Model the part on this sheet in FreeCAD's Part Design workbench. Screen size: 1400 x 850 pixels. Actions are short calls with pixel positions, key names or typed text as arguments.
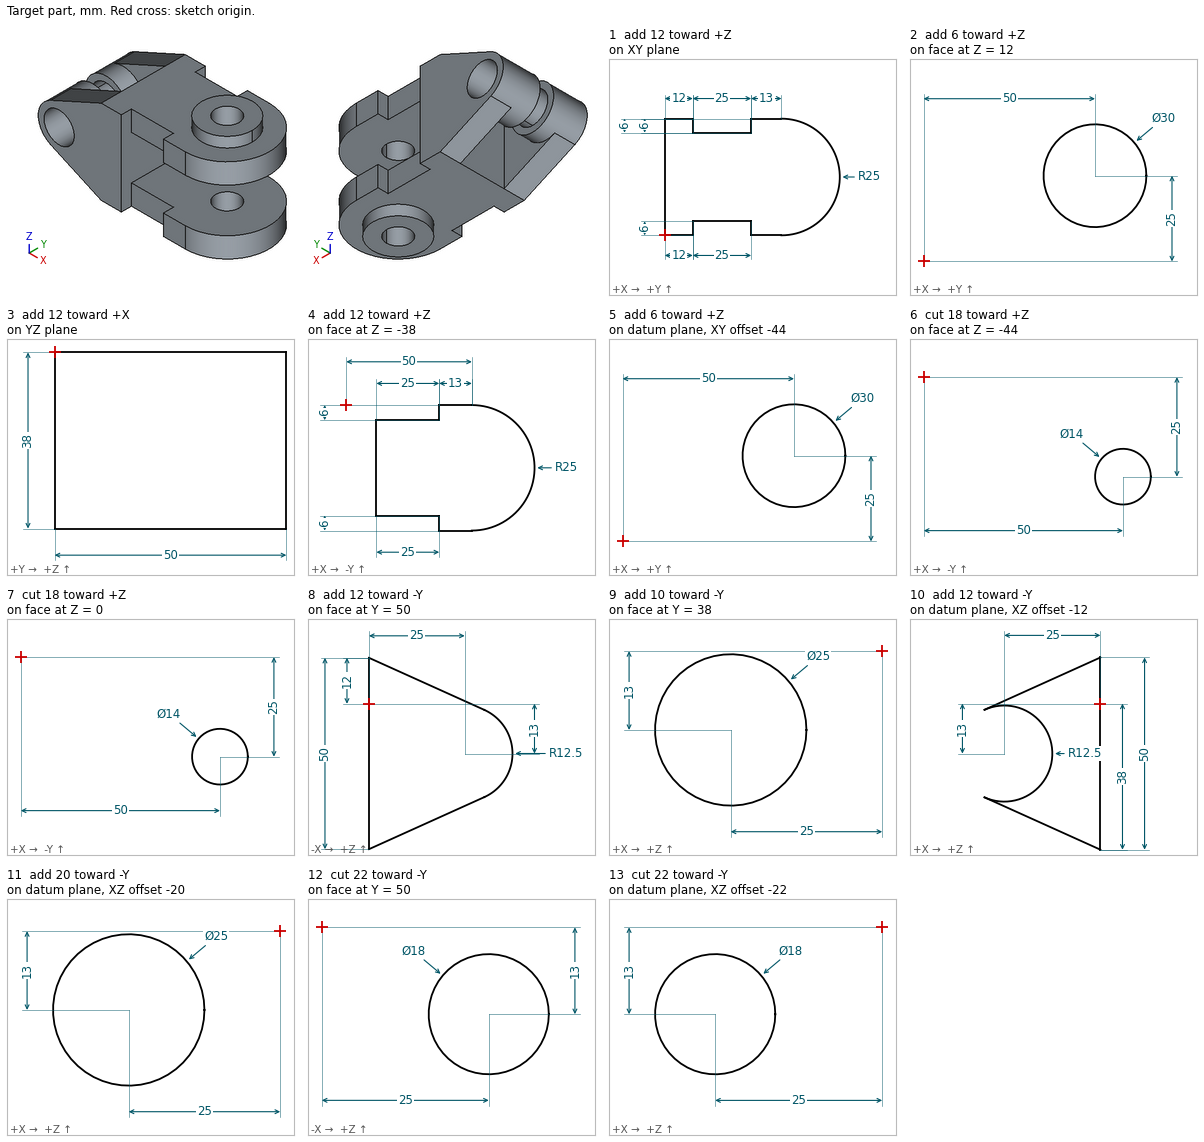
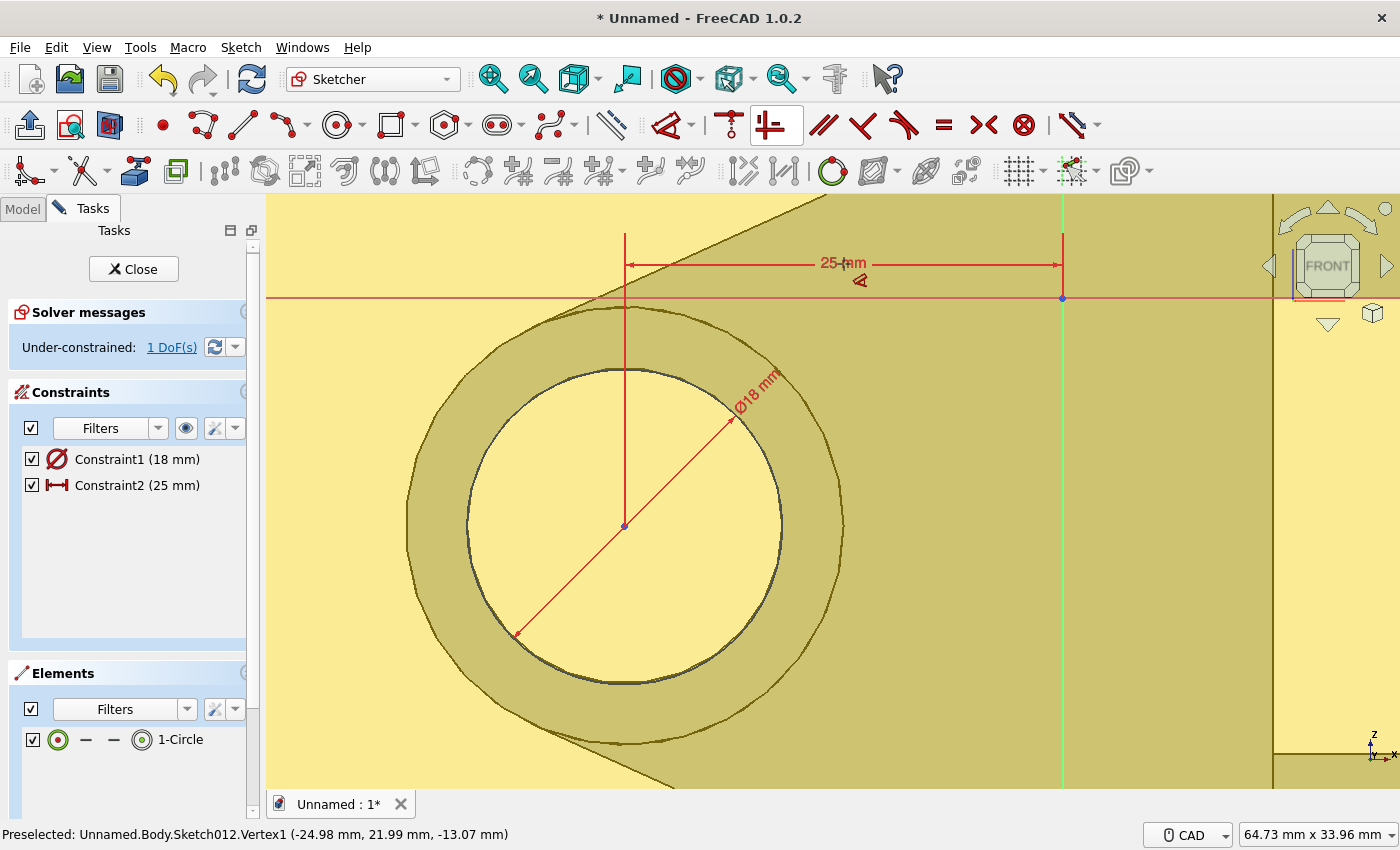
click(625, 527)
click(1097, 413)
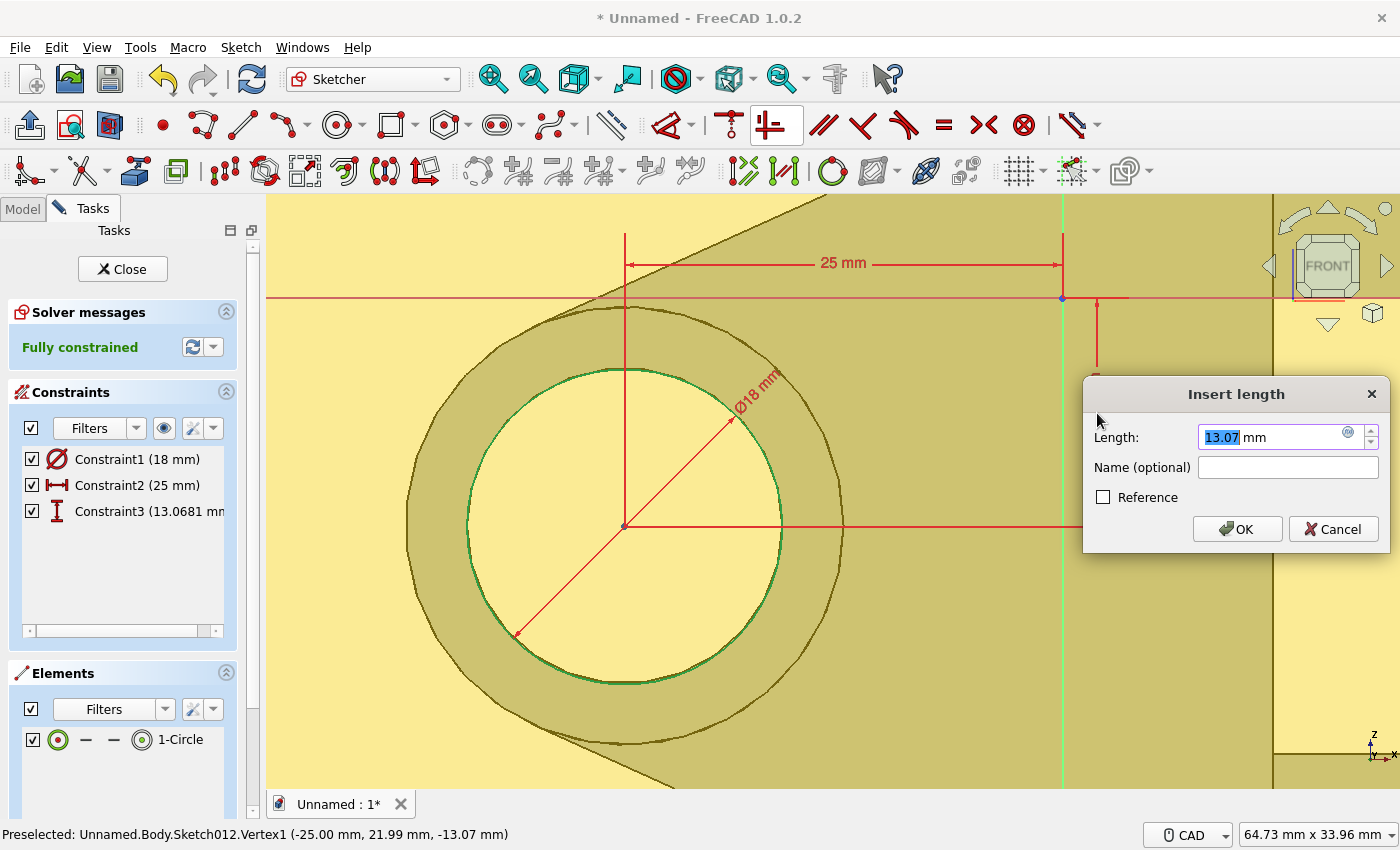
text(13)
key(Return)
key(Escape)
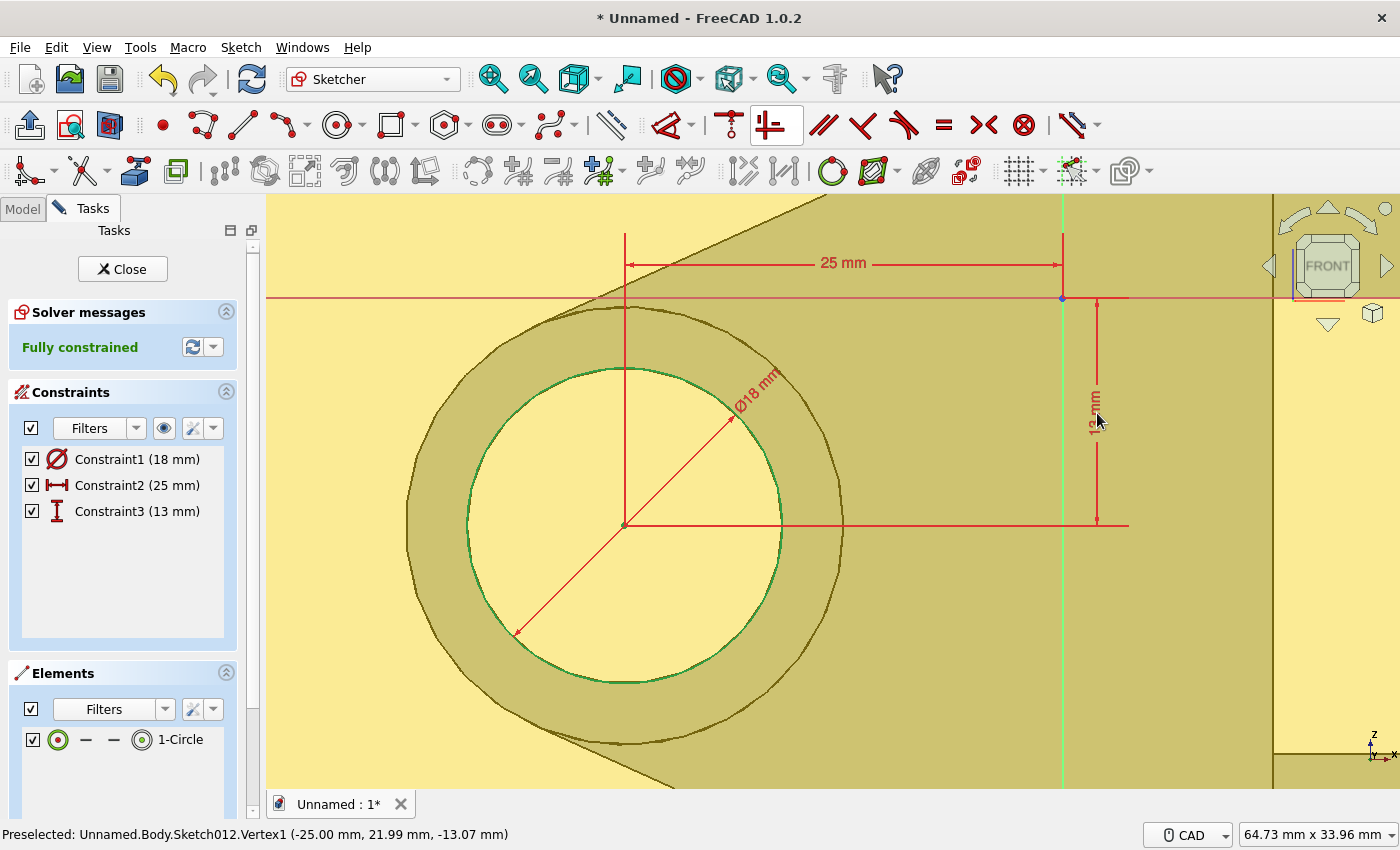
click(123, 269)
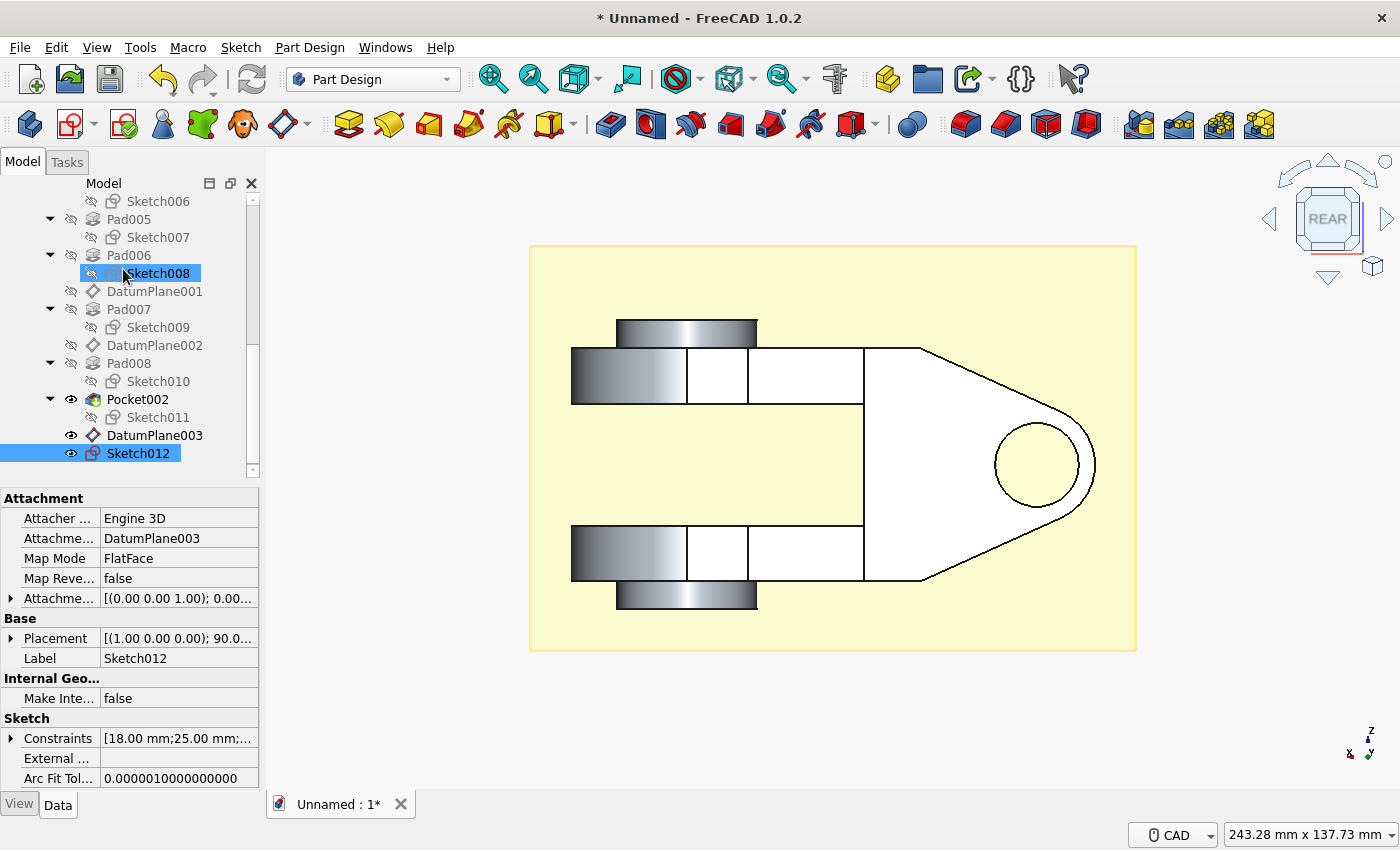
click(612, 124)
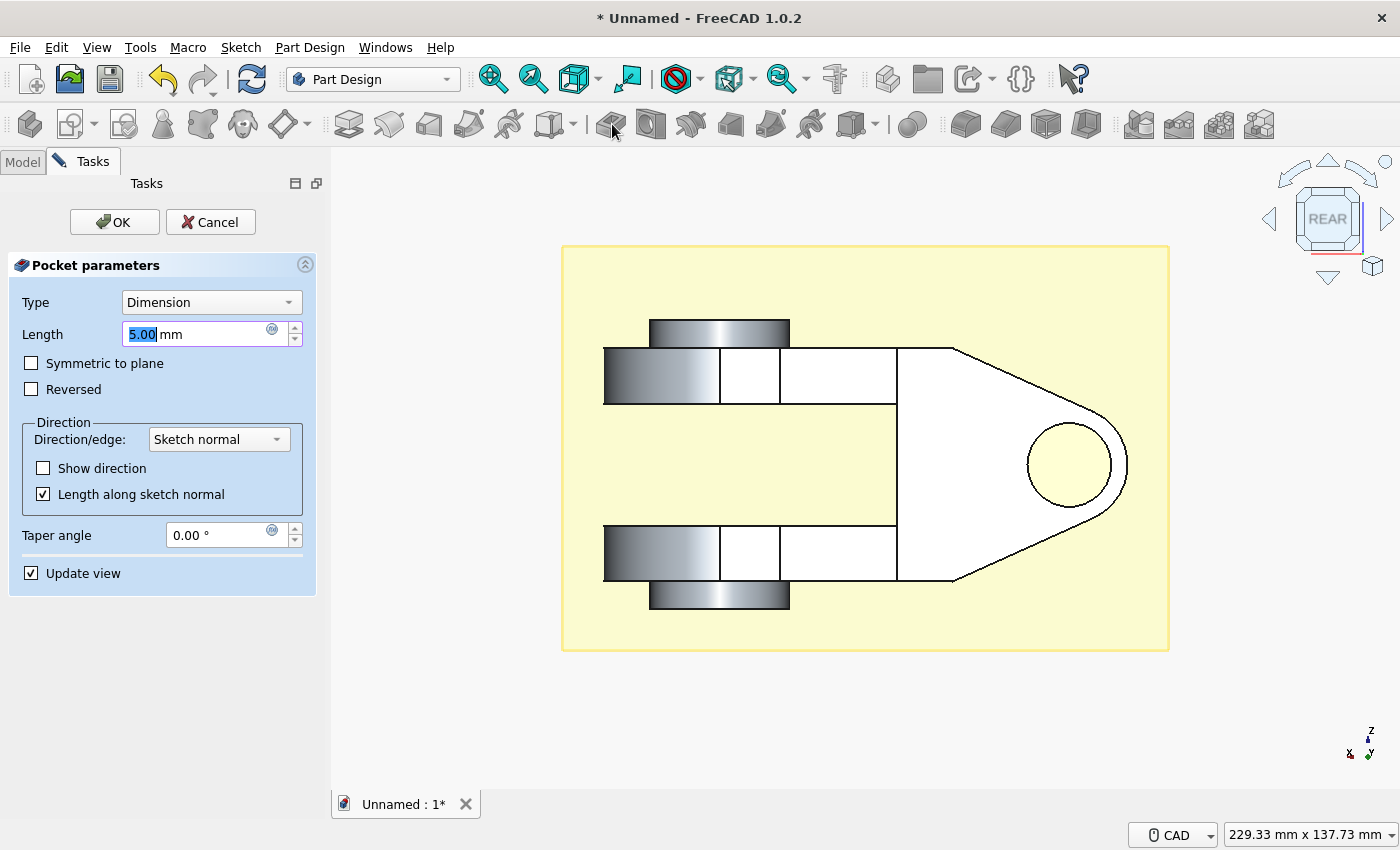
text(22)
key(Tab)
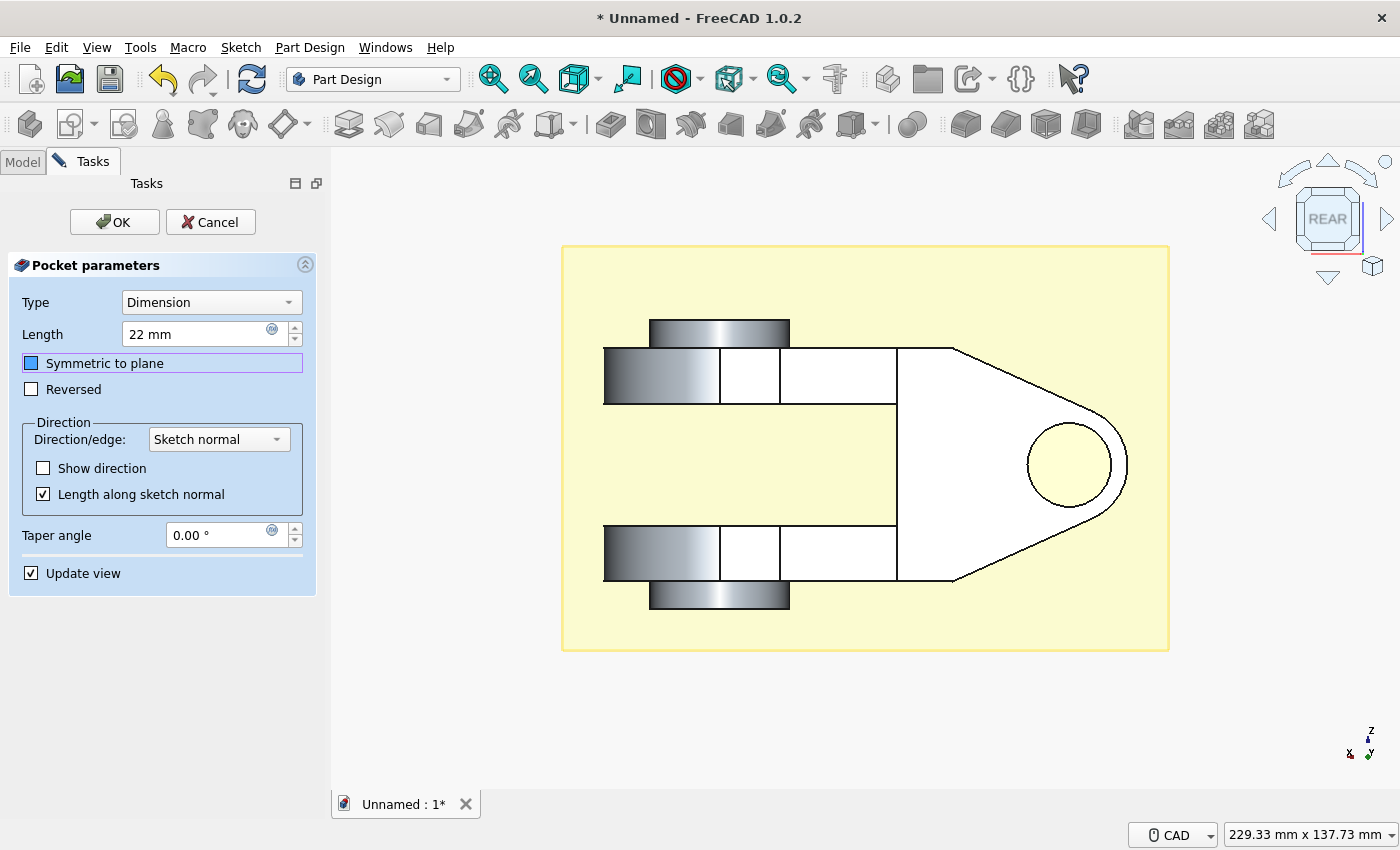
click(30, 389)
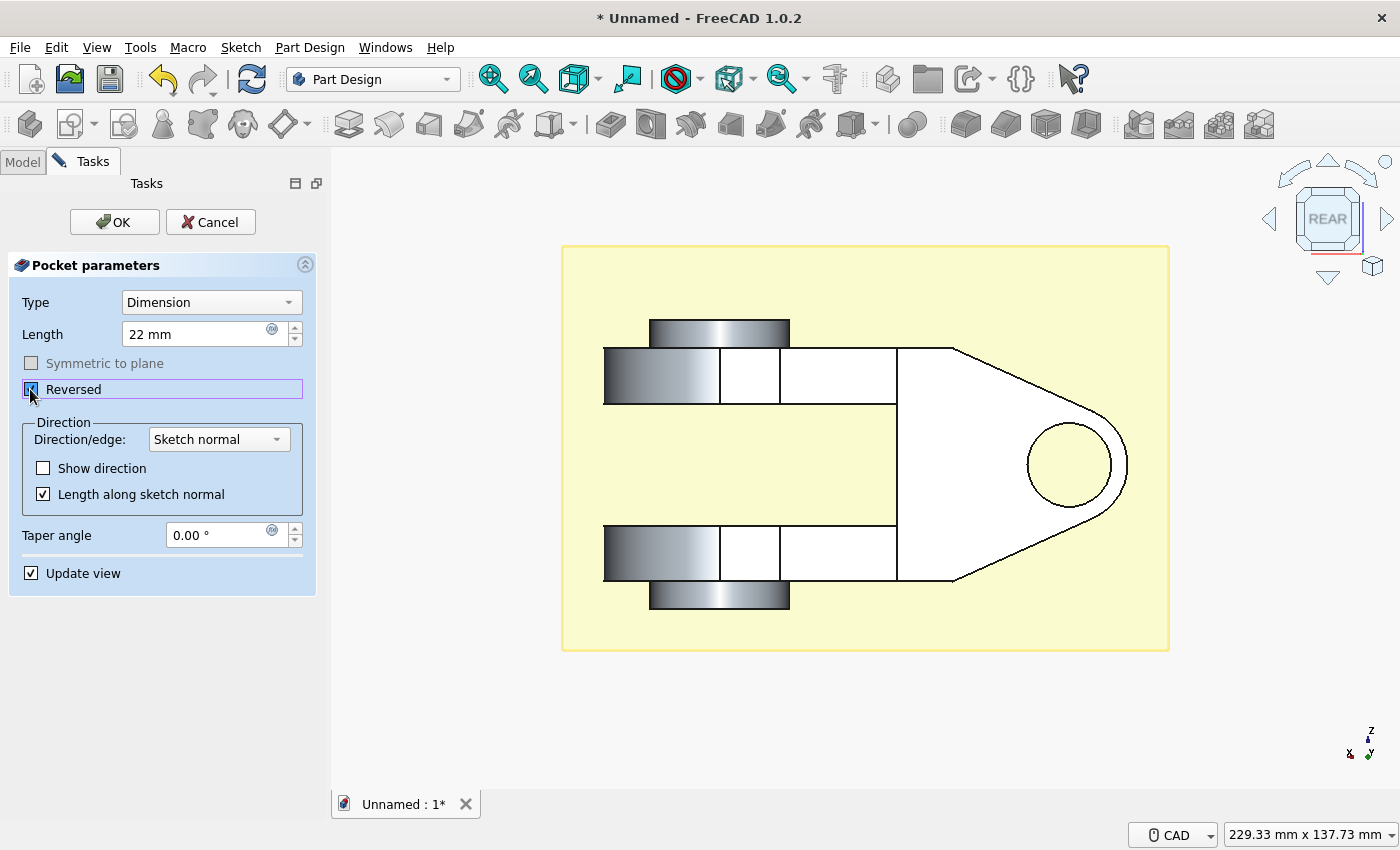
click(115, 222)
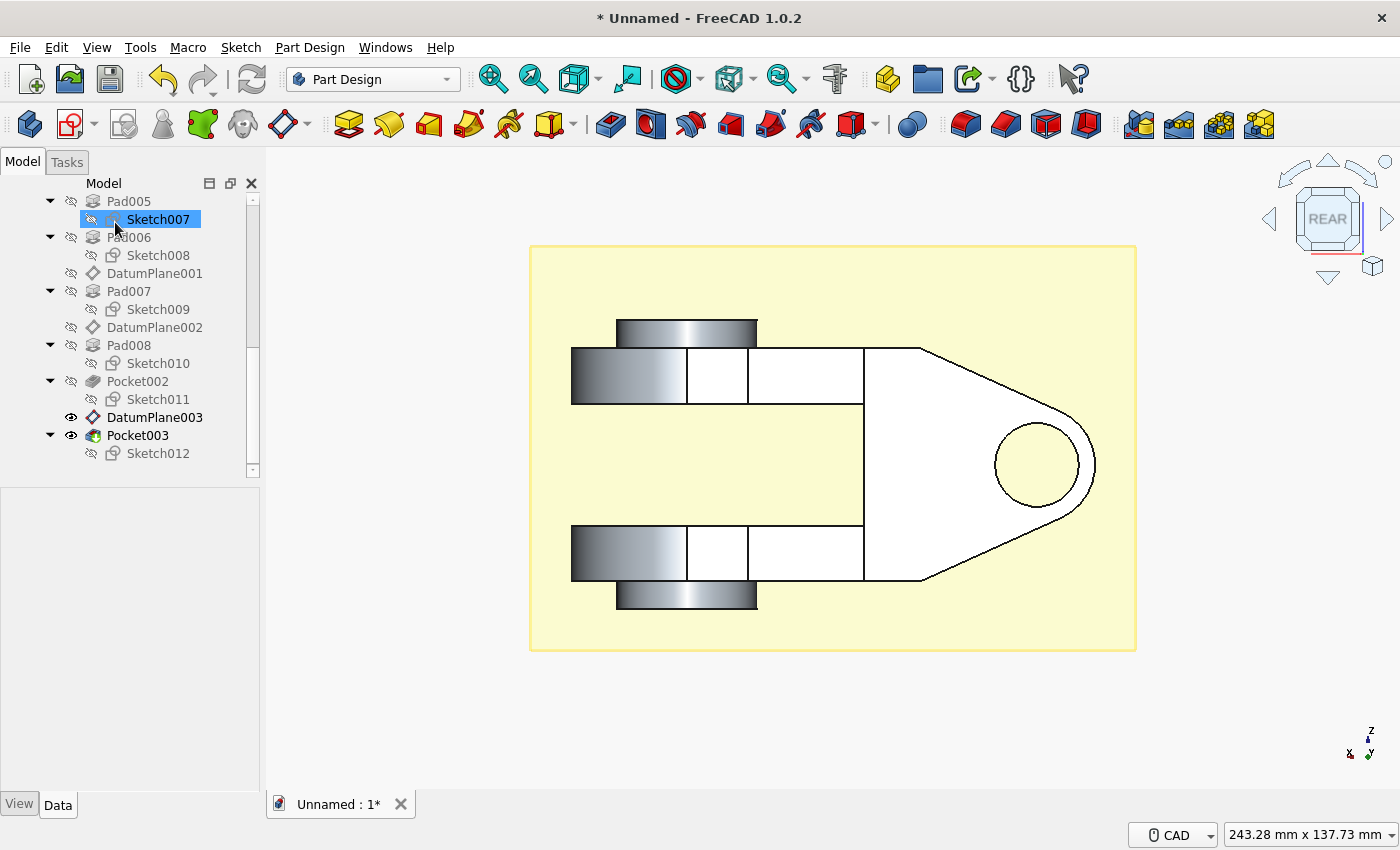
click(116, 417)
key(space)